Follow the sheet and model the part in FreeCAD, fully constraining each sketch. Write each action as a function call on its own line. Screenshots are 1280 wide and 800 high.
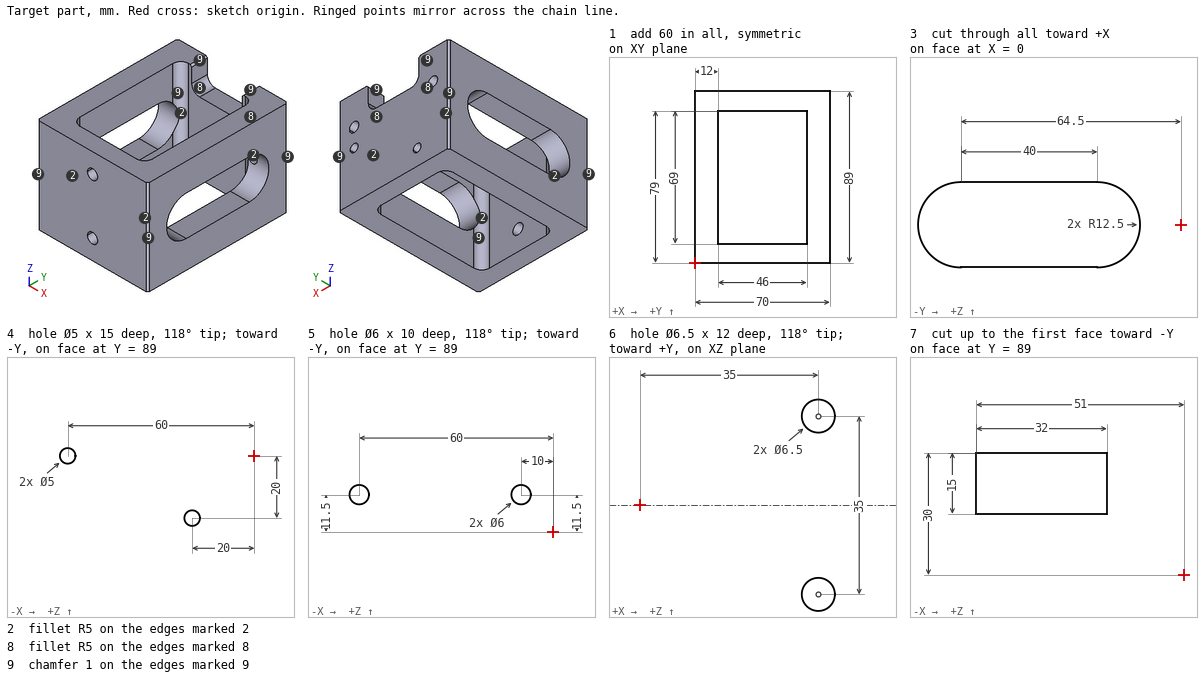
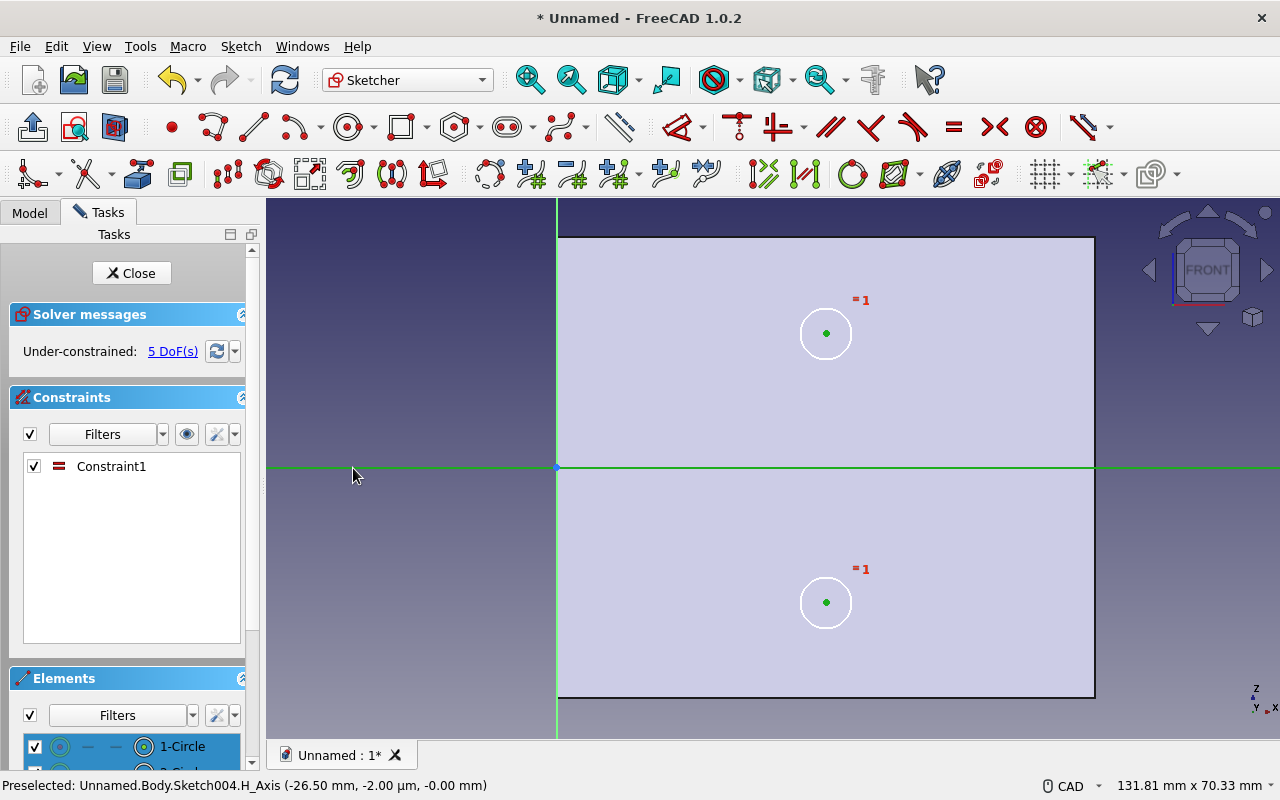
click(995, 128)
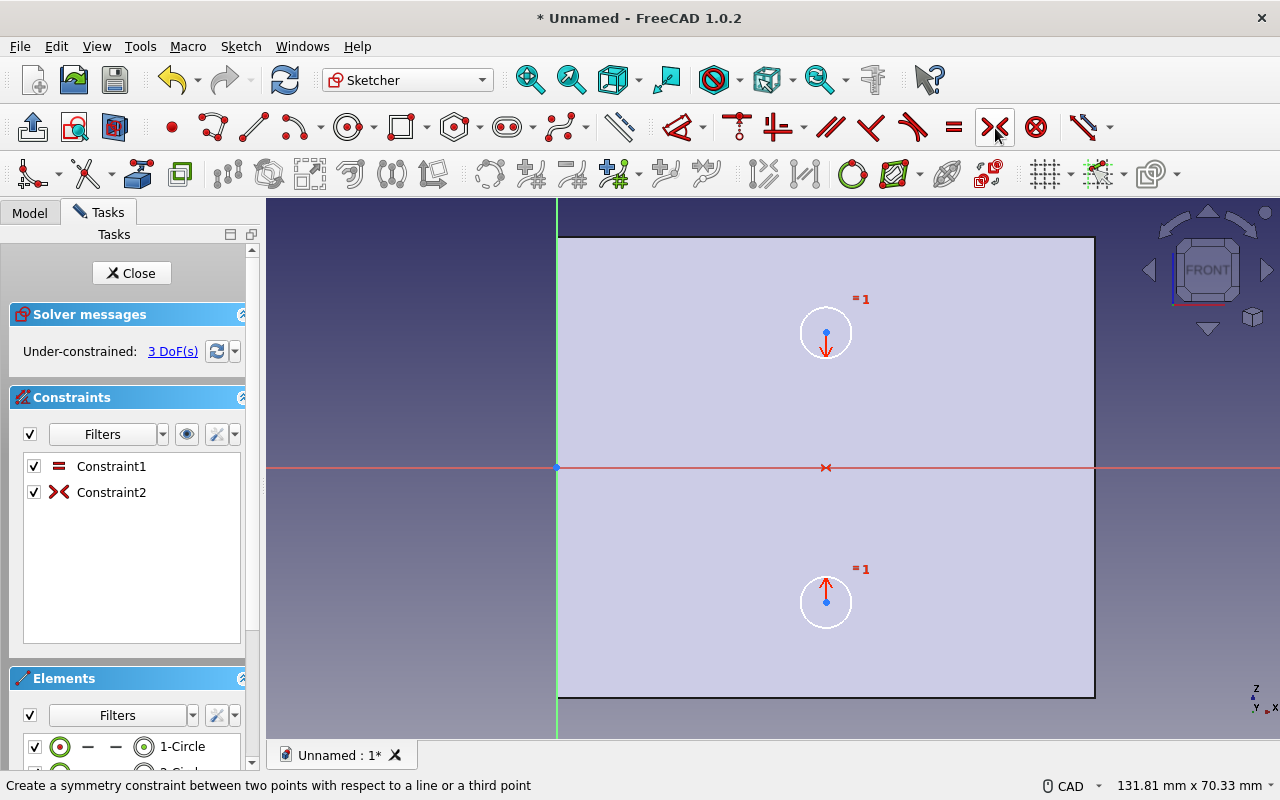
click(676, 128)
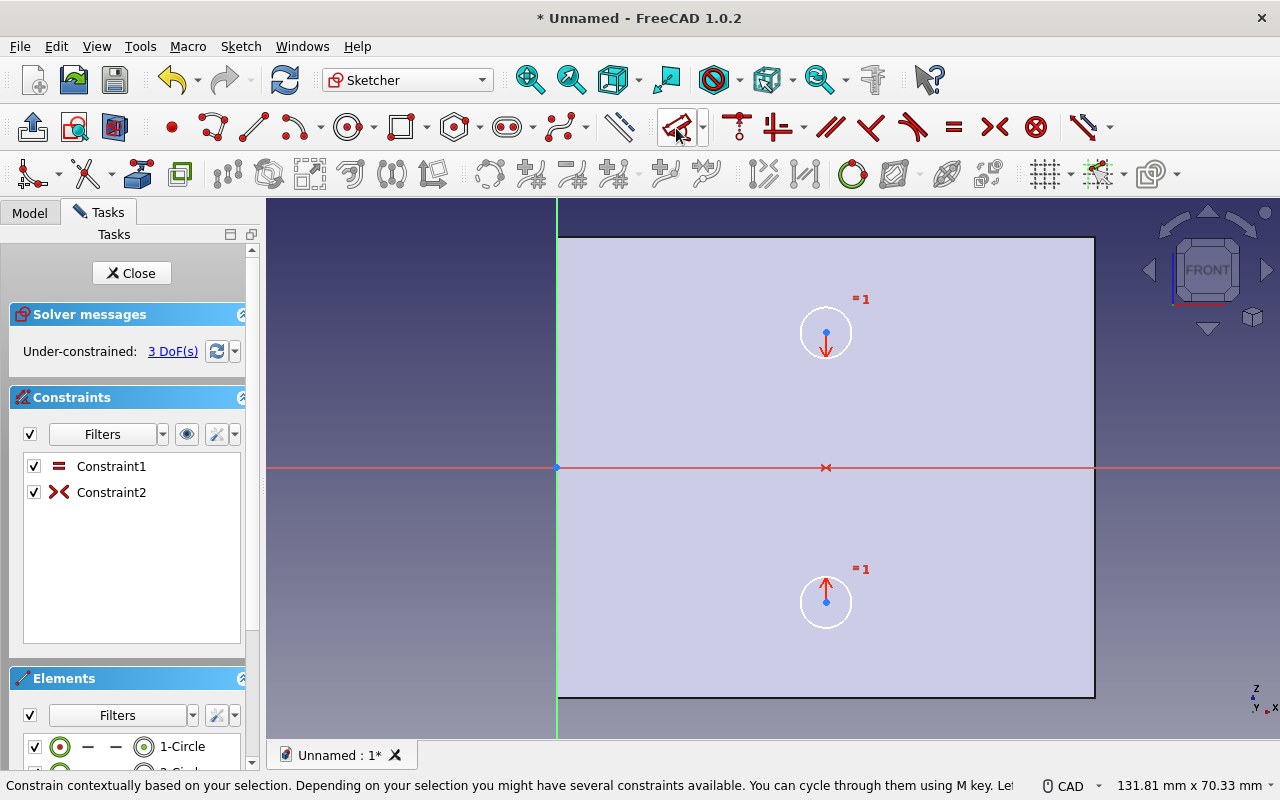
click(844, 315)
click(867, 292)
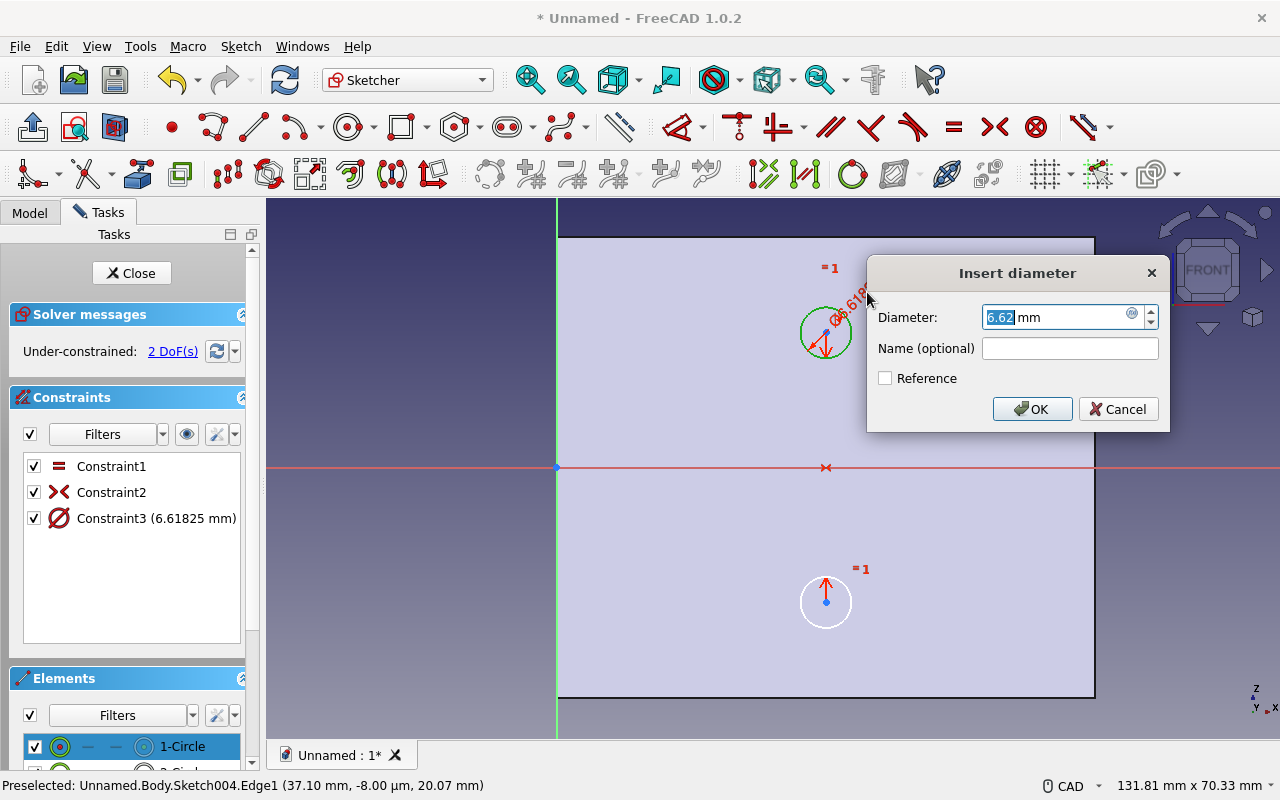
text(6.5)
key(Return)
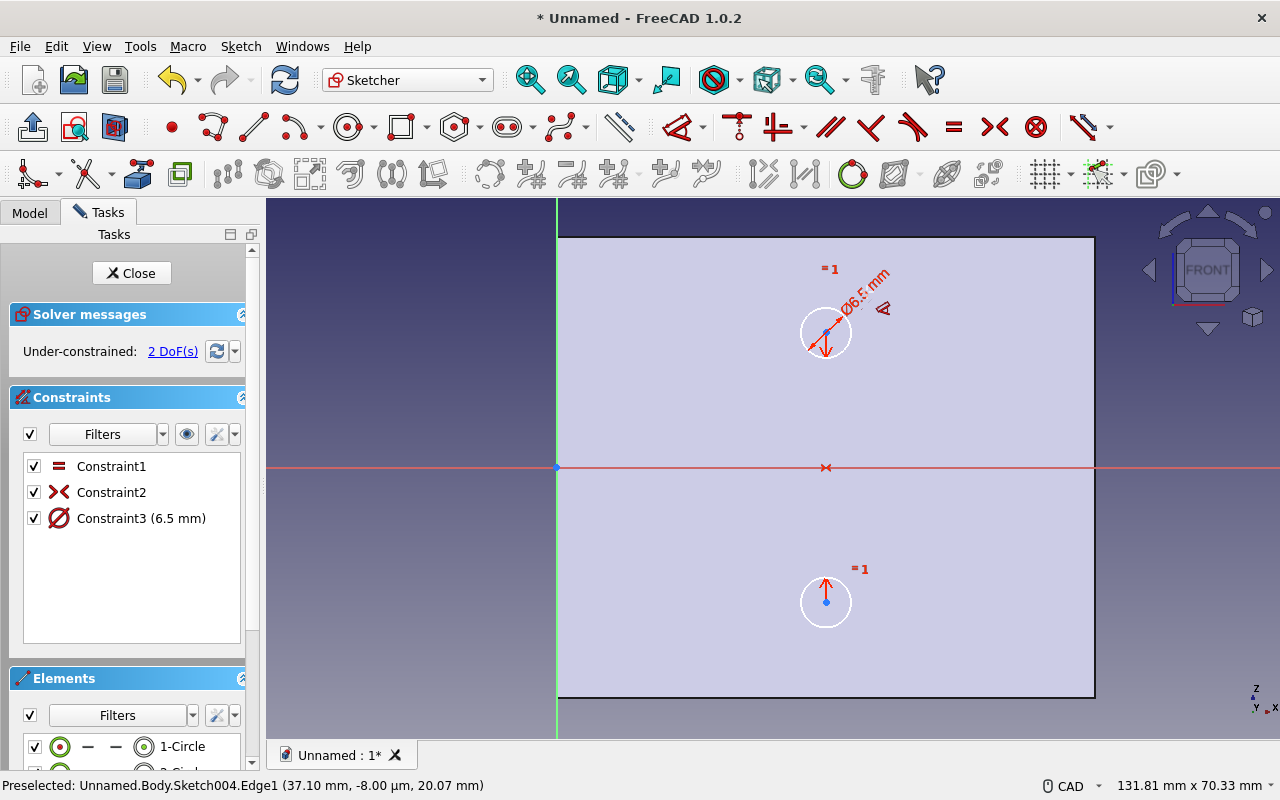
click(826, 333)
click(691, 299)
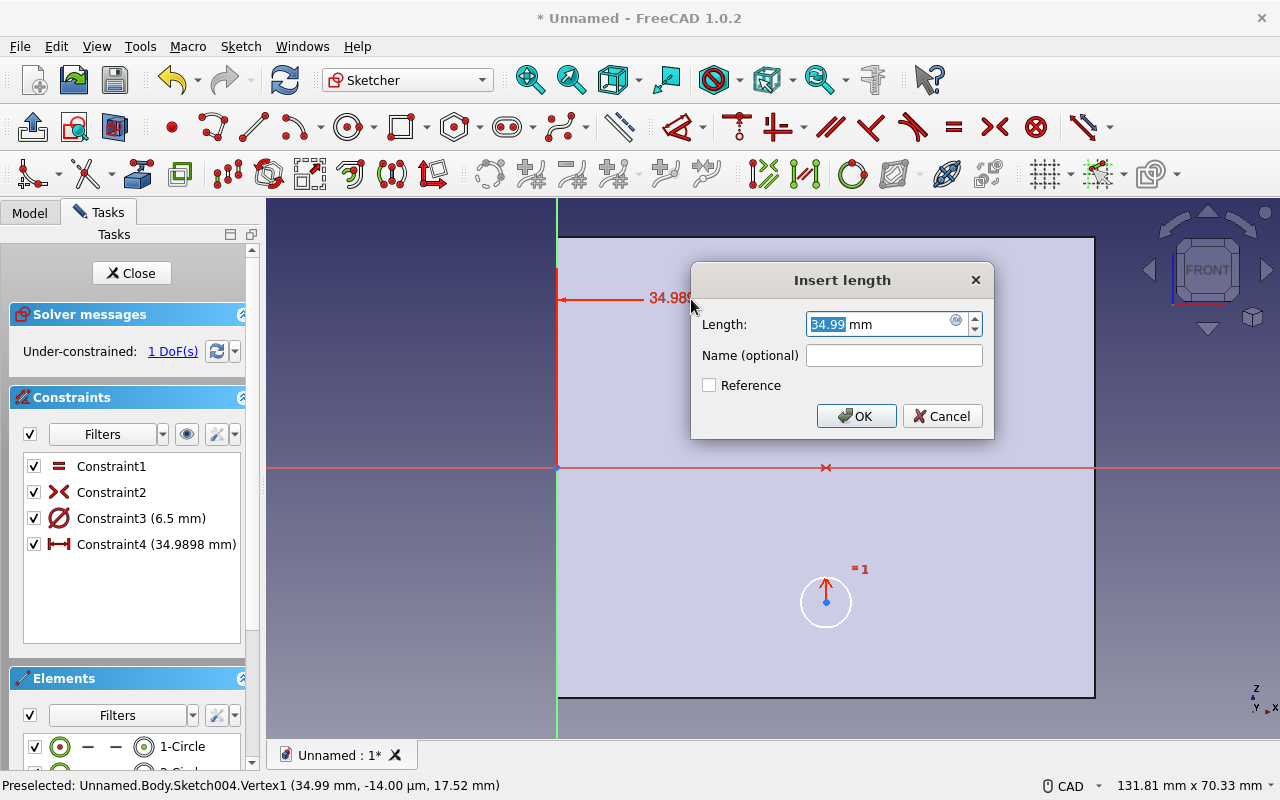
text(35)
key(Return)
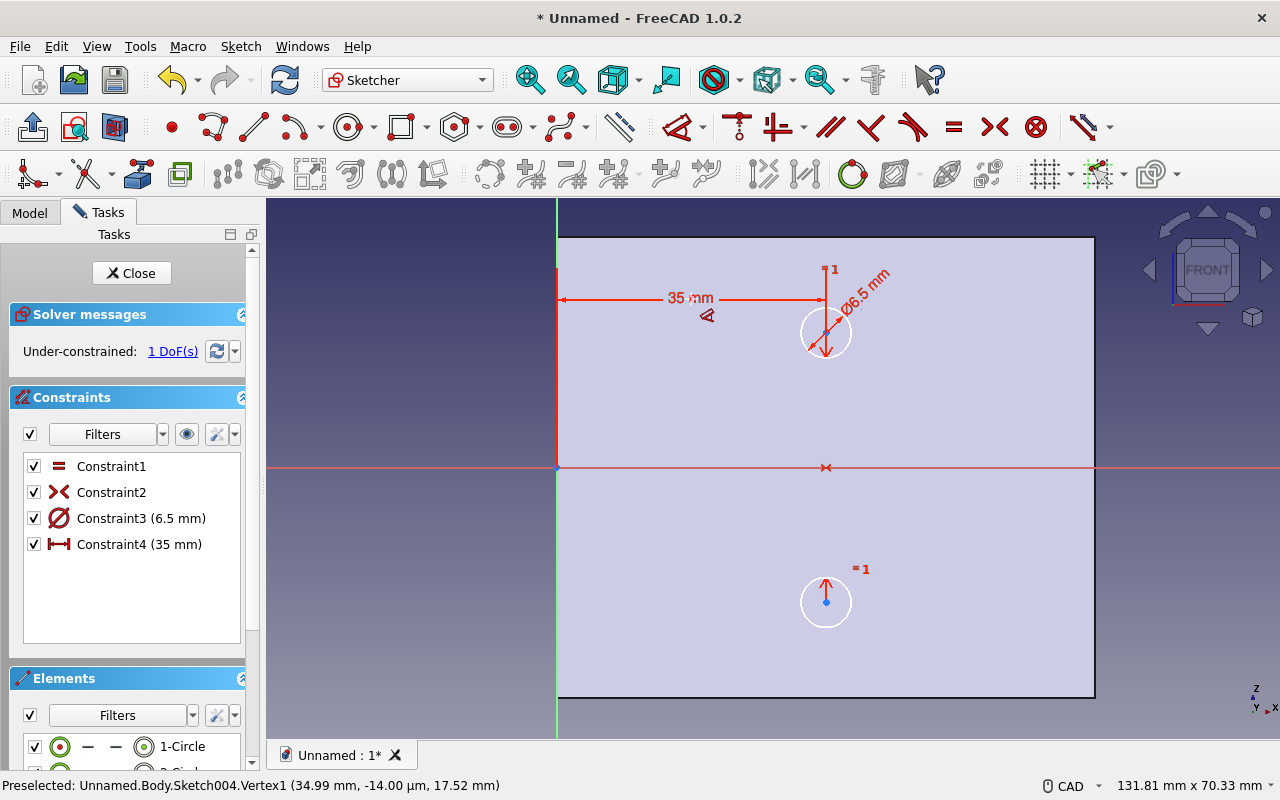
click(826, 333)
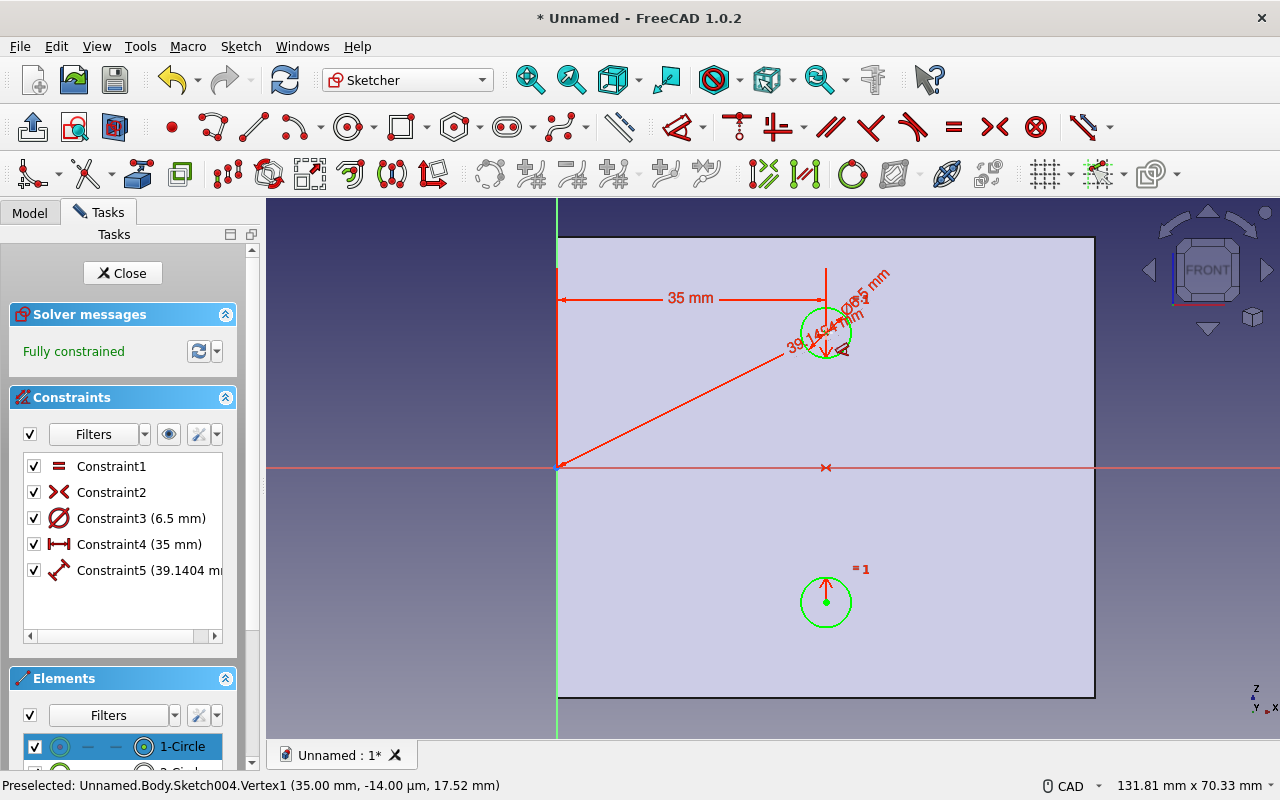
click(826, 602)
click(860, 406)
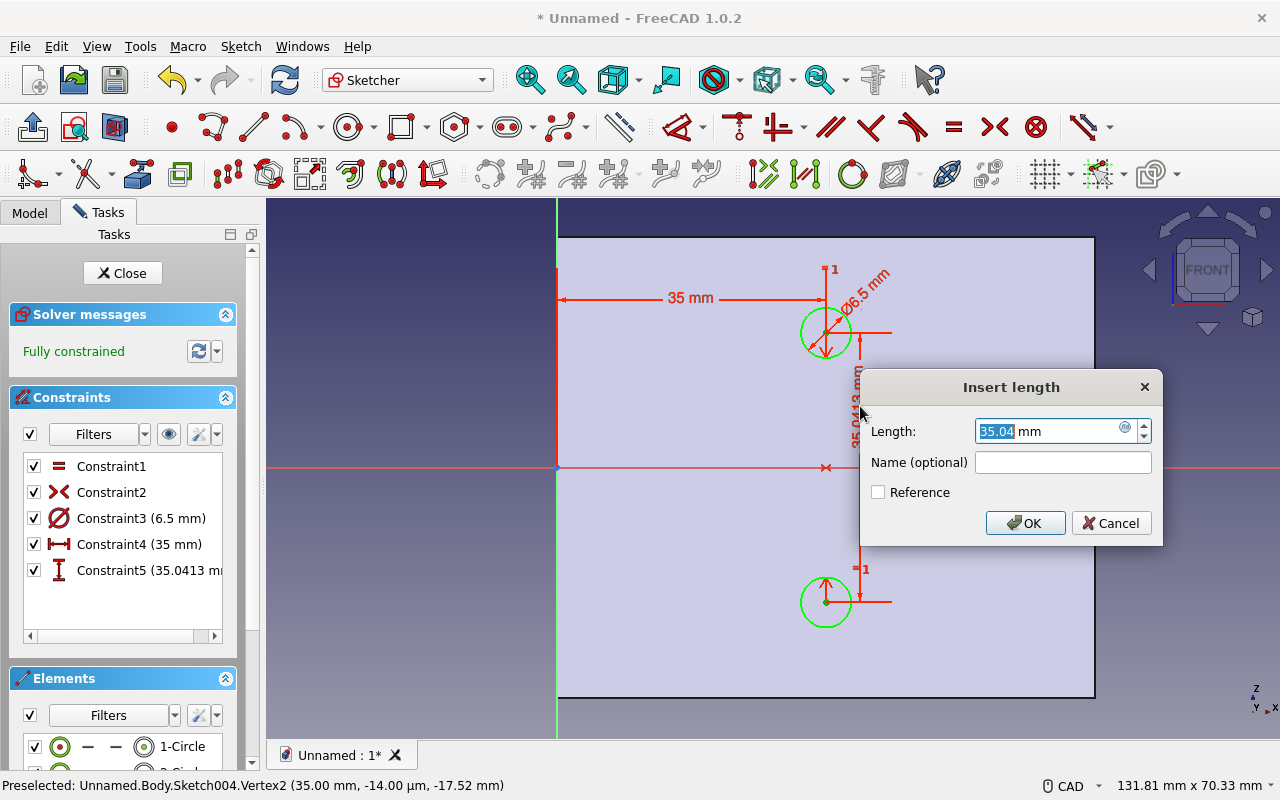
text(35)
key(Return)
key(Escape)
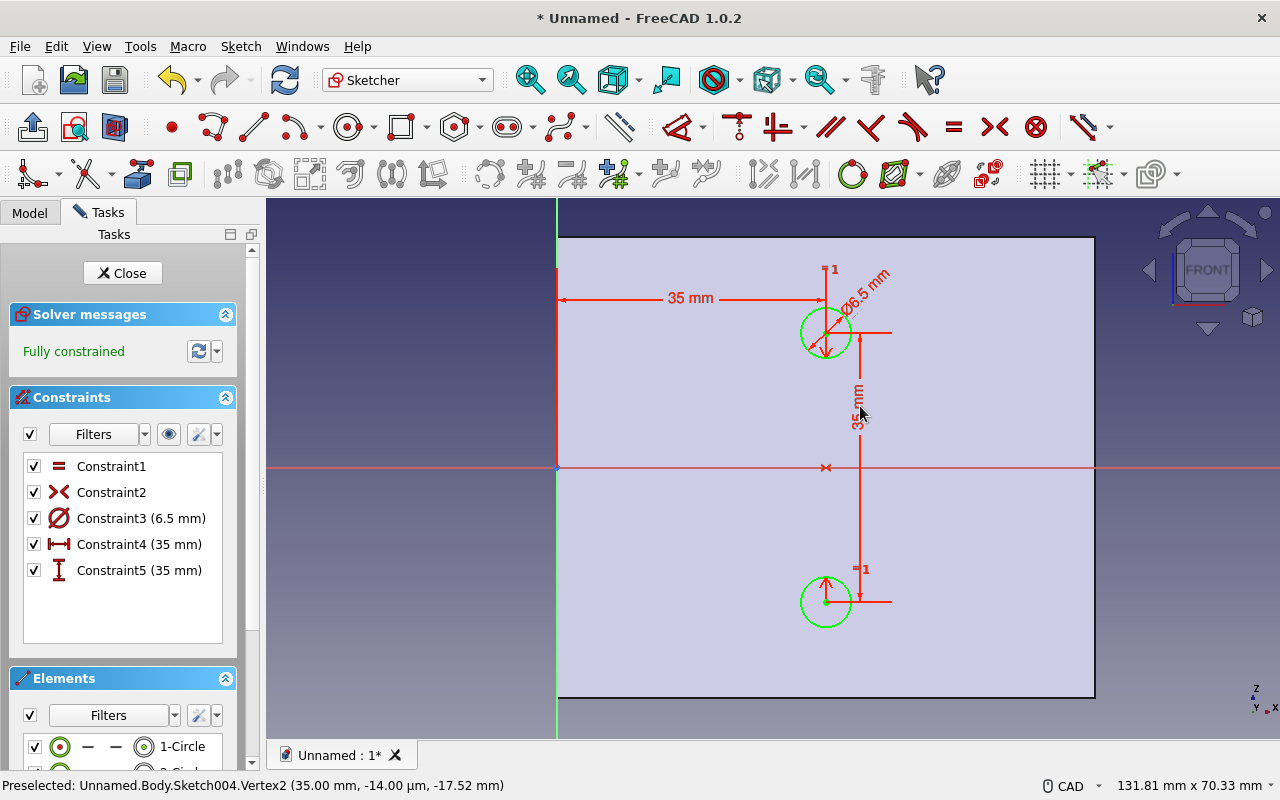
click(123, 273)